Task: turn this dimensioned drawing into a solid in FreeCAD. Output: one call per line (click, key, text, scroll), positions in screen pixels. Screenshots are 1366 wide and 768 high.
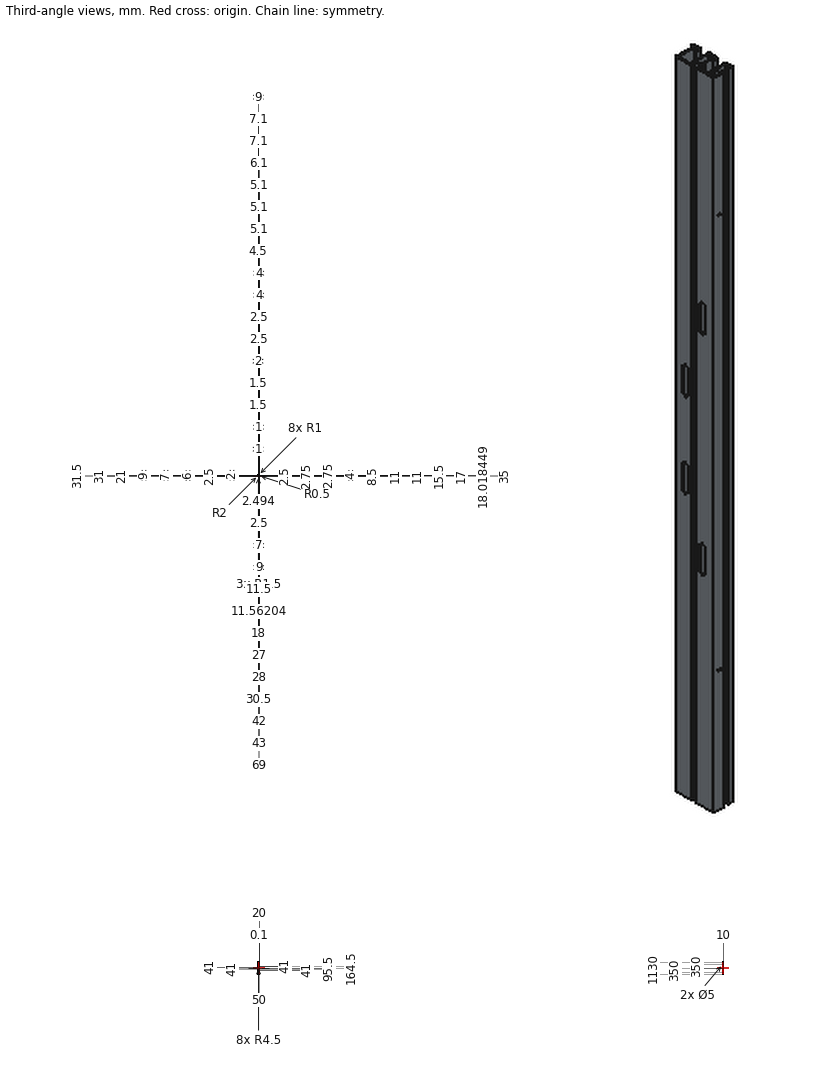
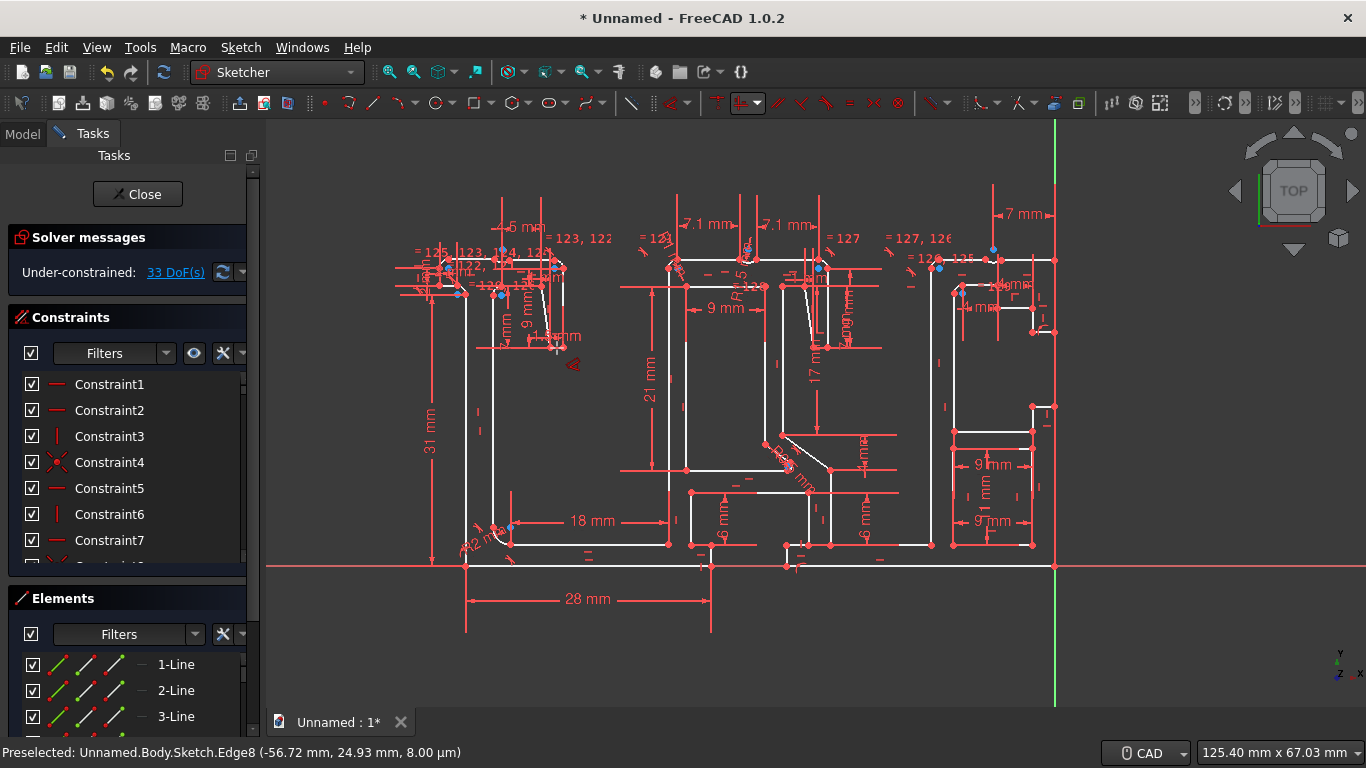
click(541, 260)
click(532, 202)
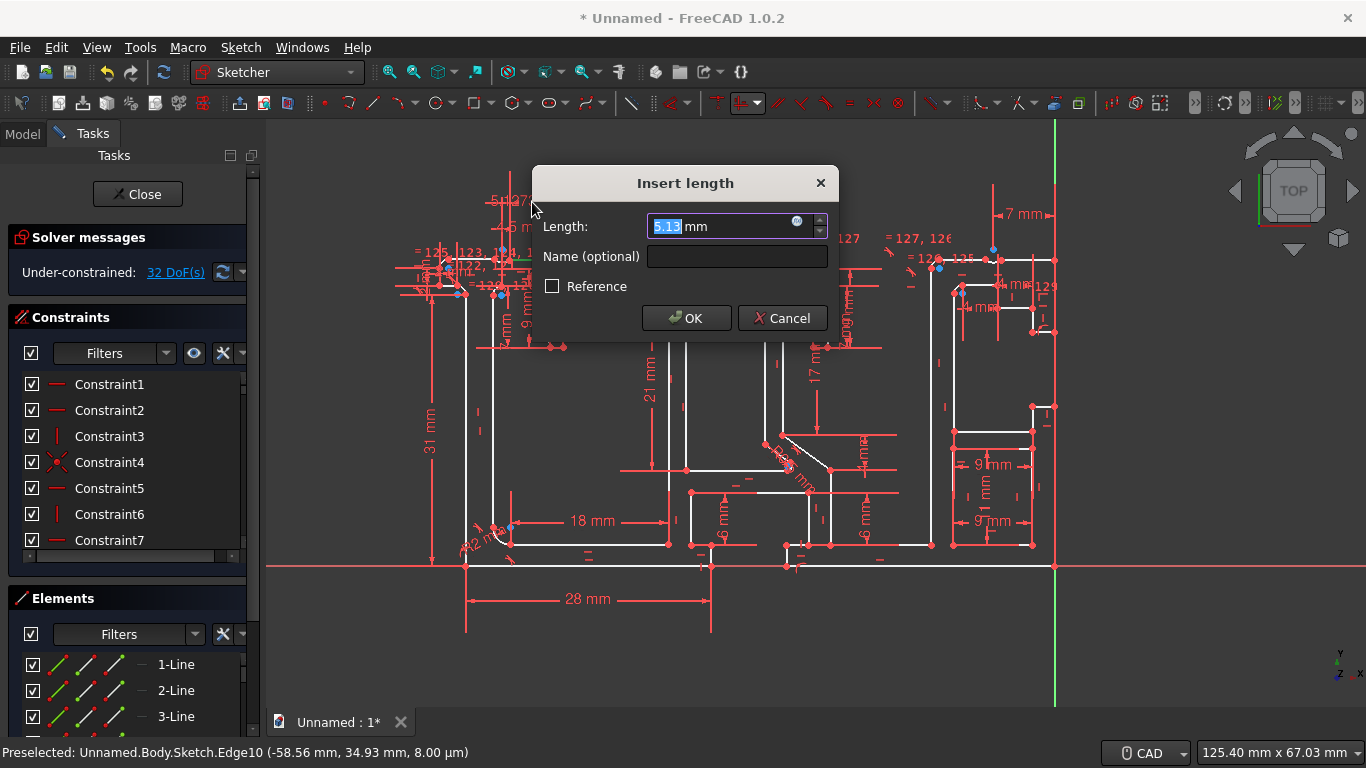
text(5.1)
key(Return)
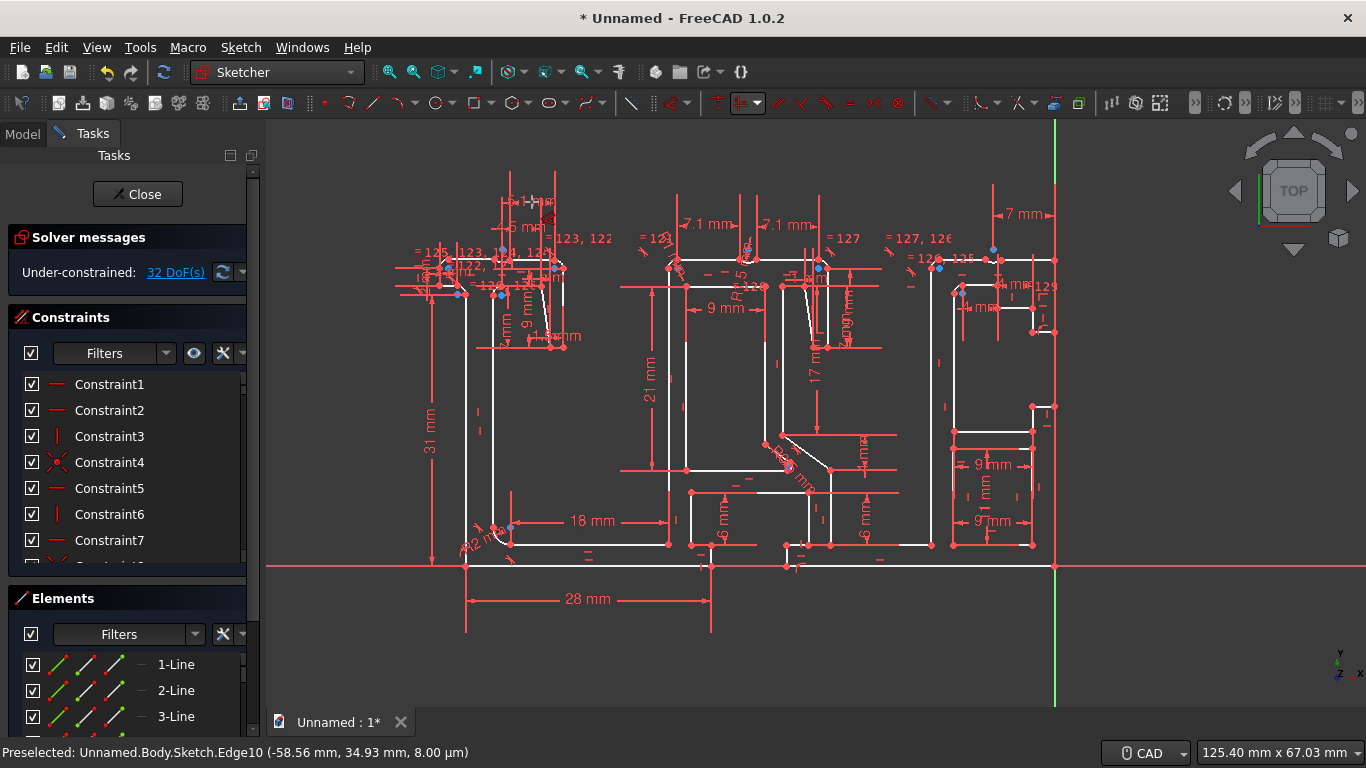
click(481, 259)
click(461, 201)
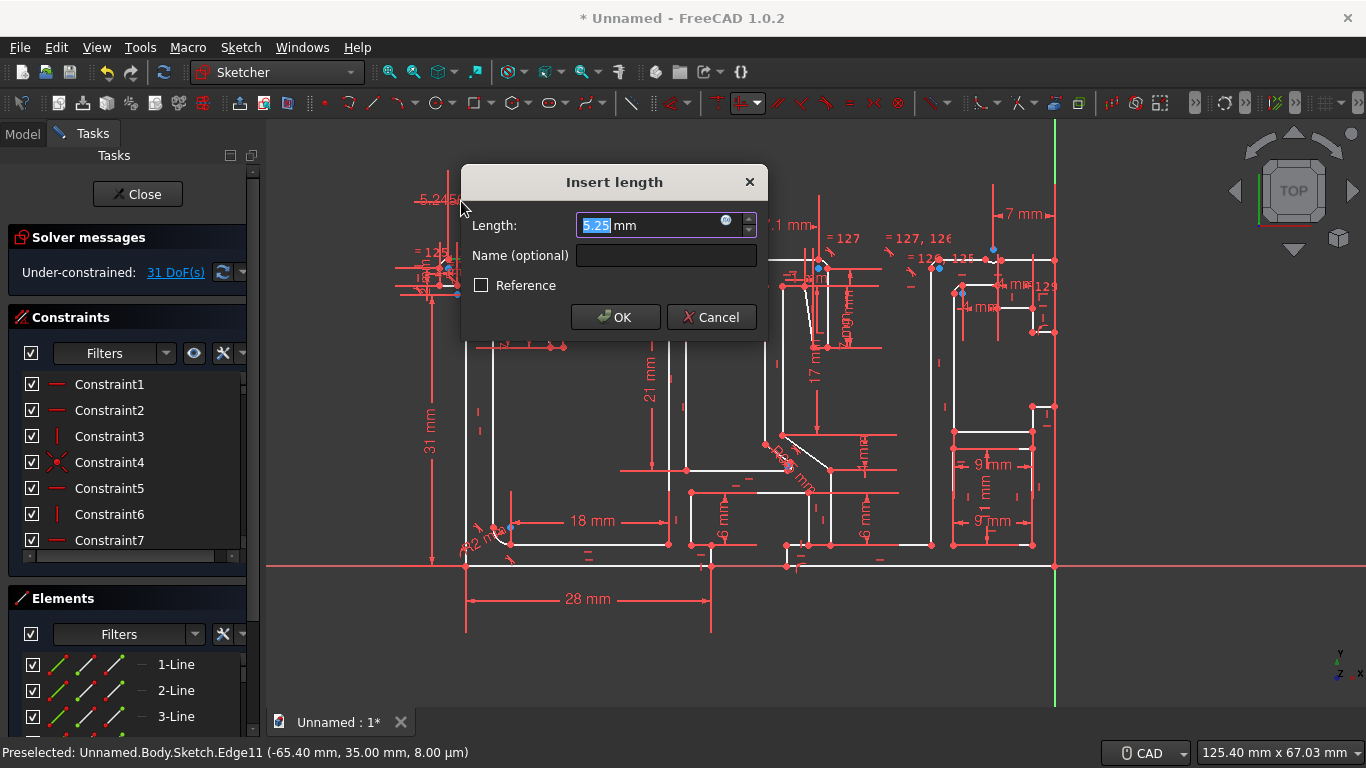
text(5.1)
key(Return)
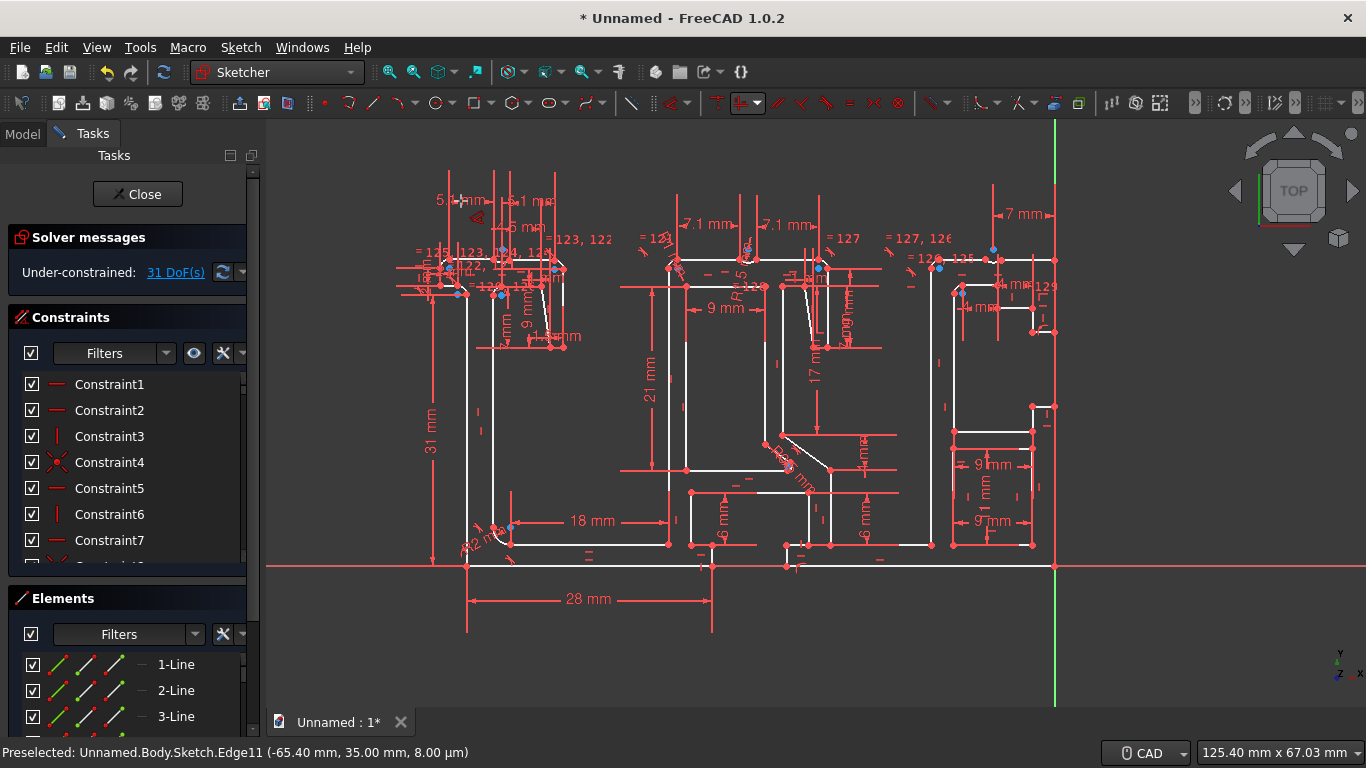
scroll(712, 556, up, 3)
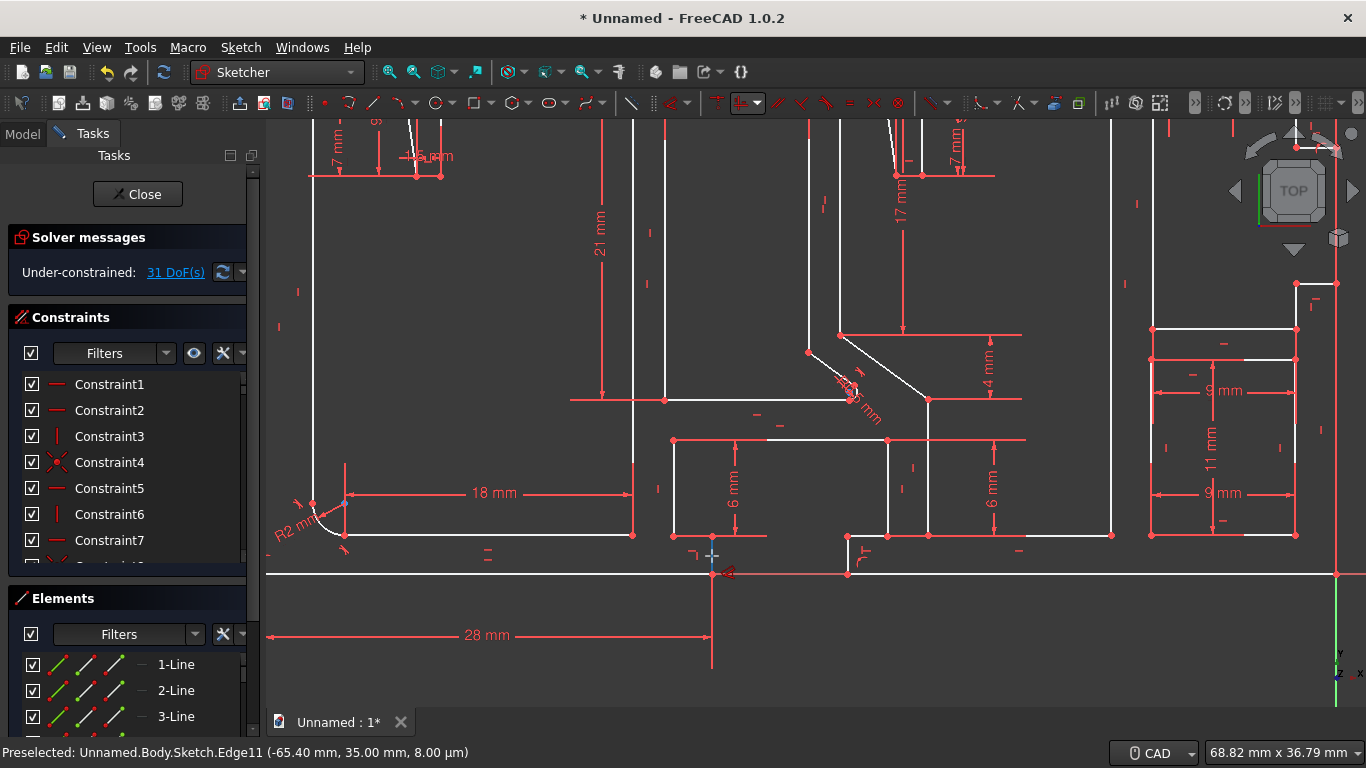
click(712, 555)
click(678, 555)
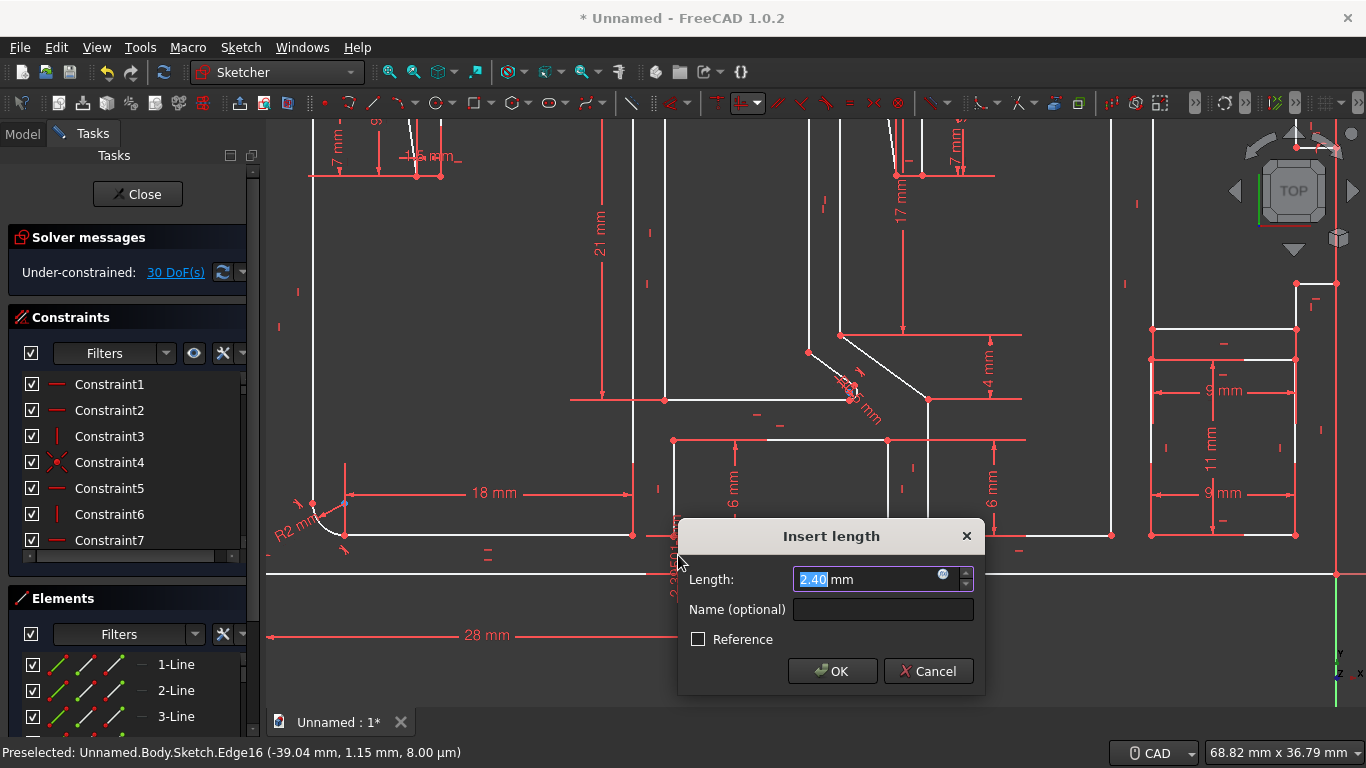
text(2.5)
key(Return)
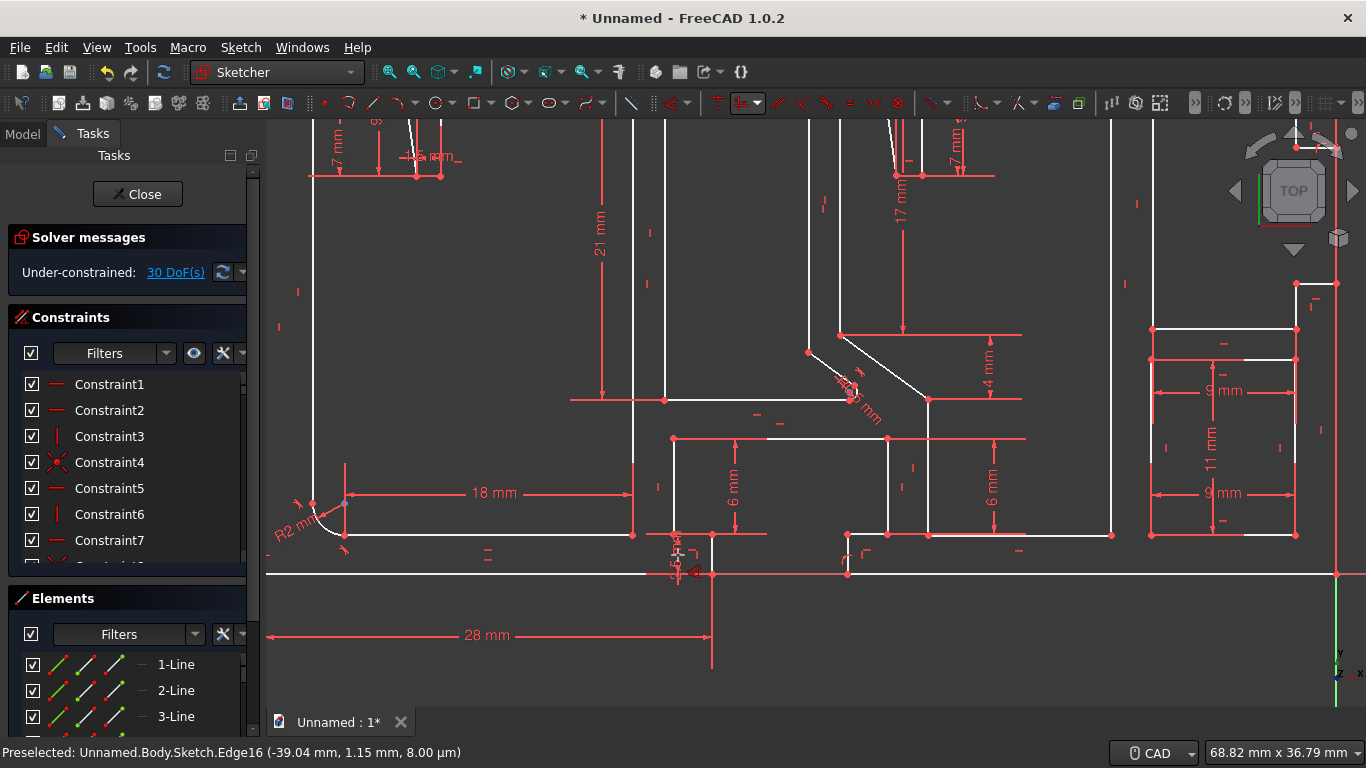
click(701, 534)
click(693, 592)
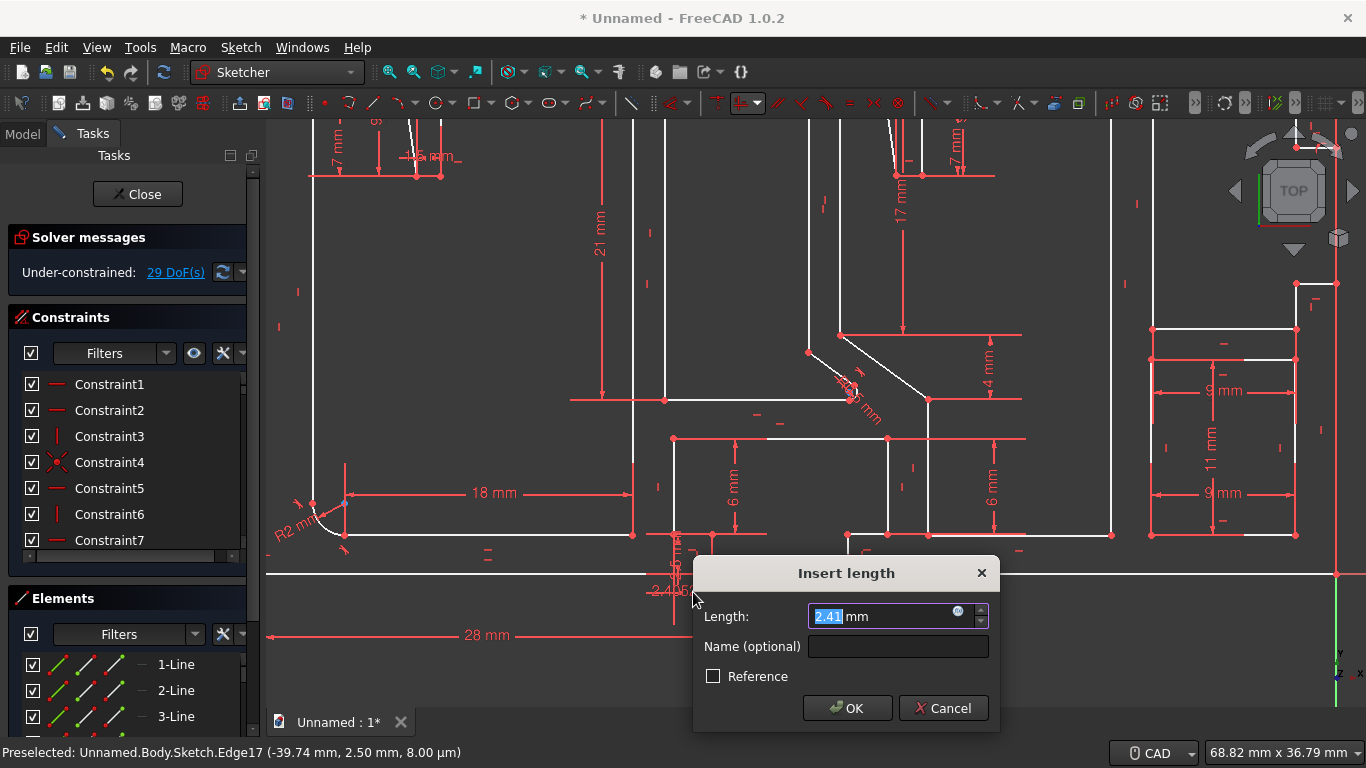
text(2.5)
key(Return)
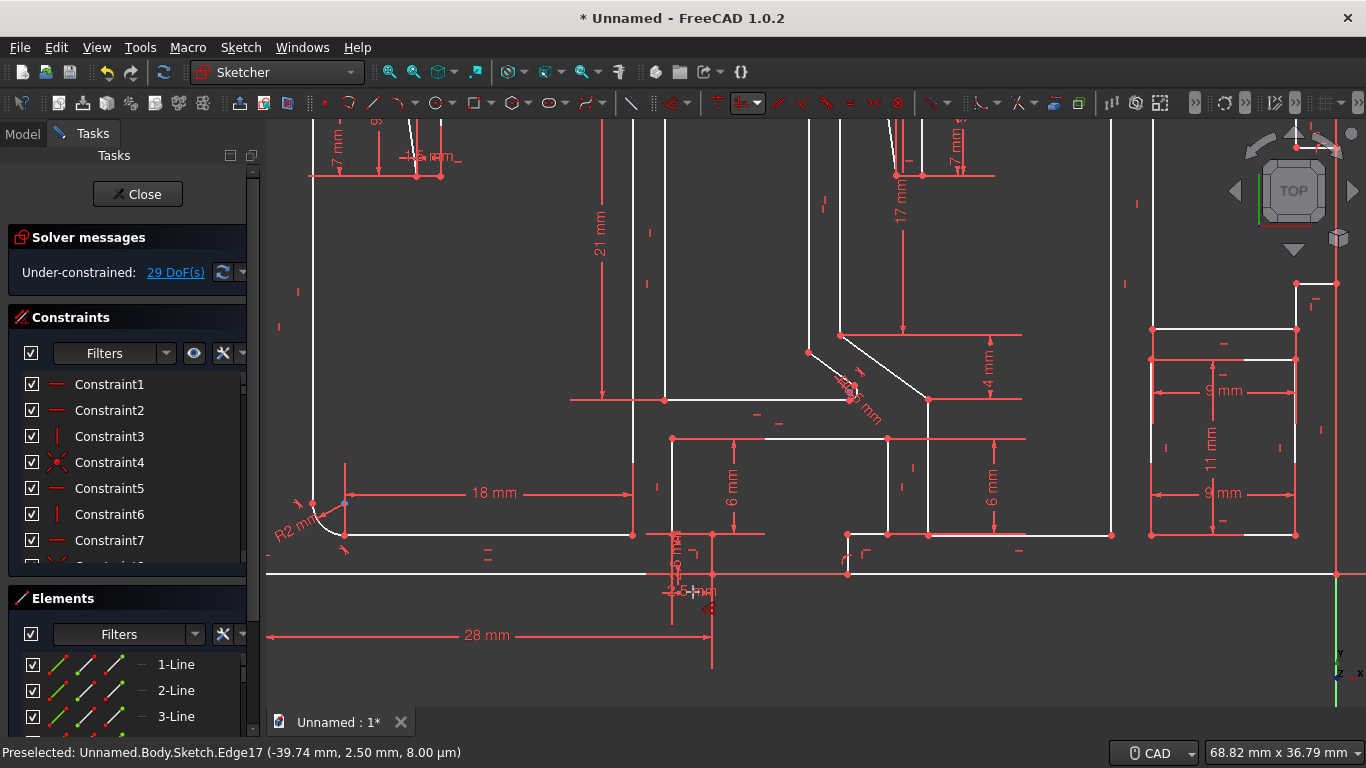
scroll(712, 557, down, 3)